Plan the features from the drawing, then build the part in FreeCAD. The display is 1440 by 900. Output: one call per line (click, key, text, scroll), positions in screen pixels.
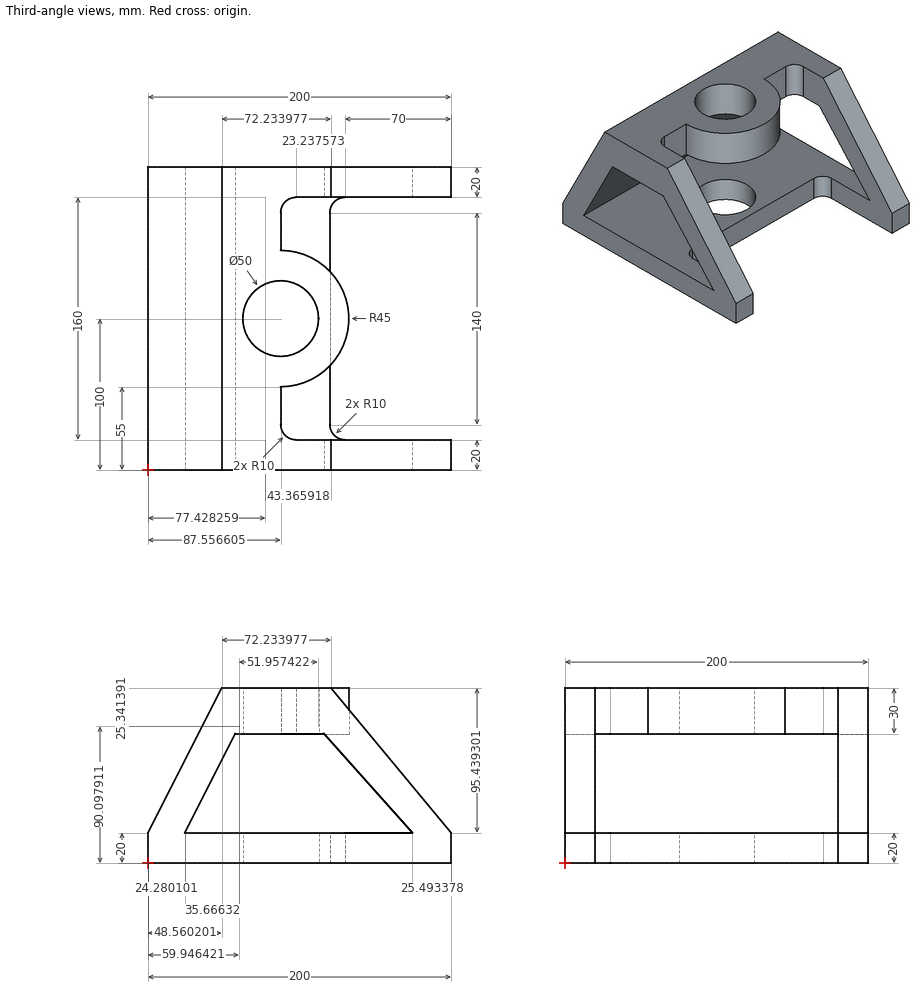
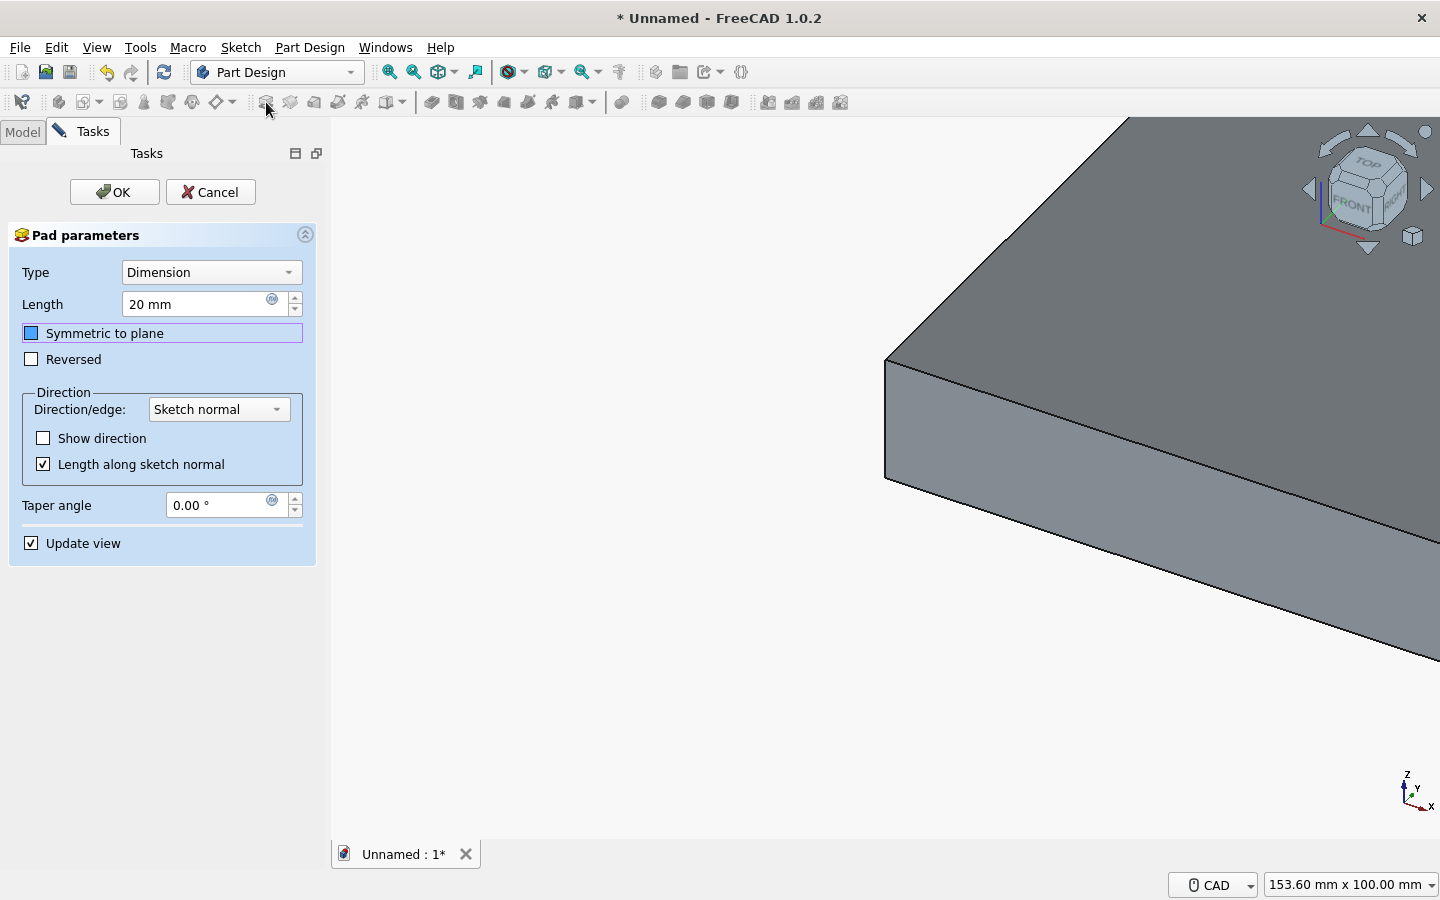
click(115, 192)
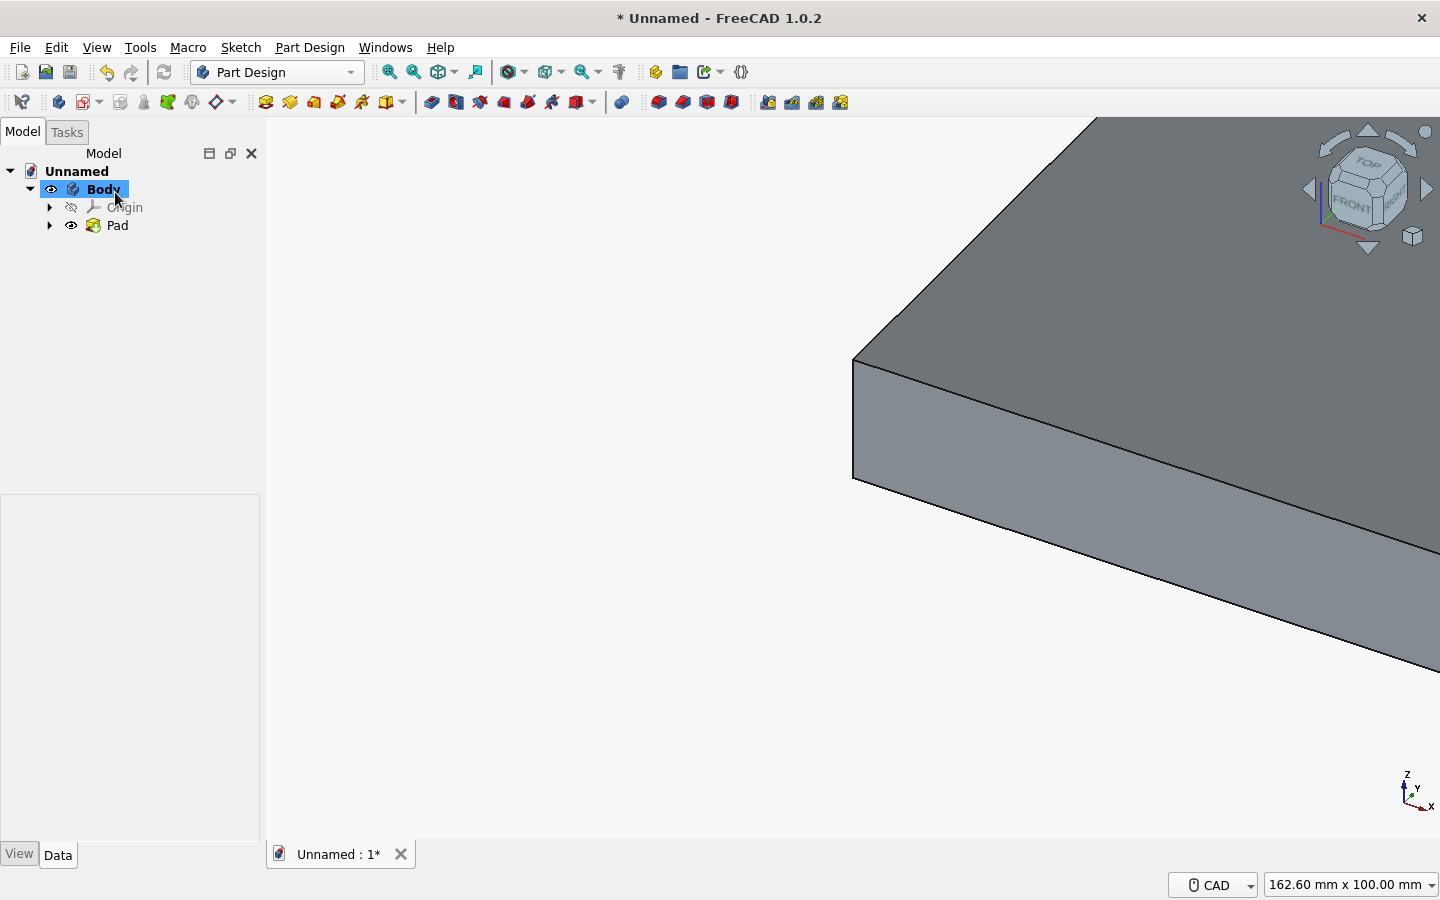
key(v)
key(f)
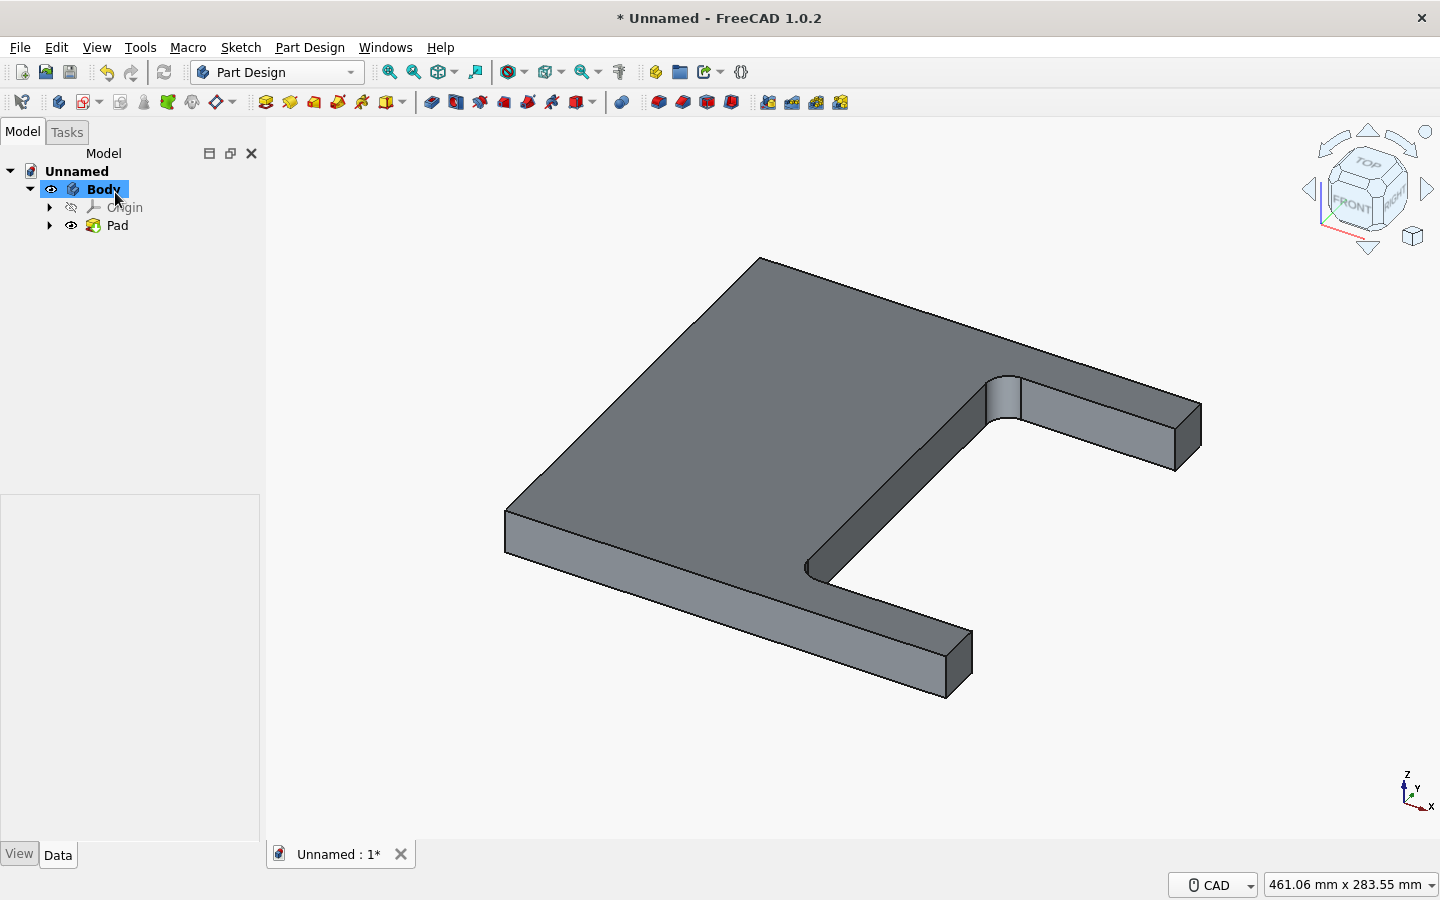
click(915, 666)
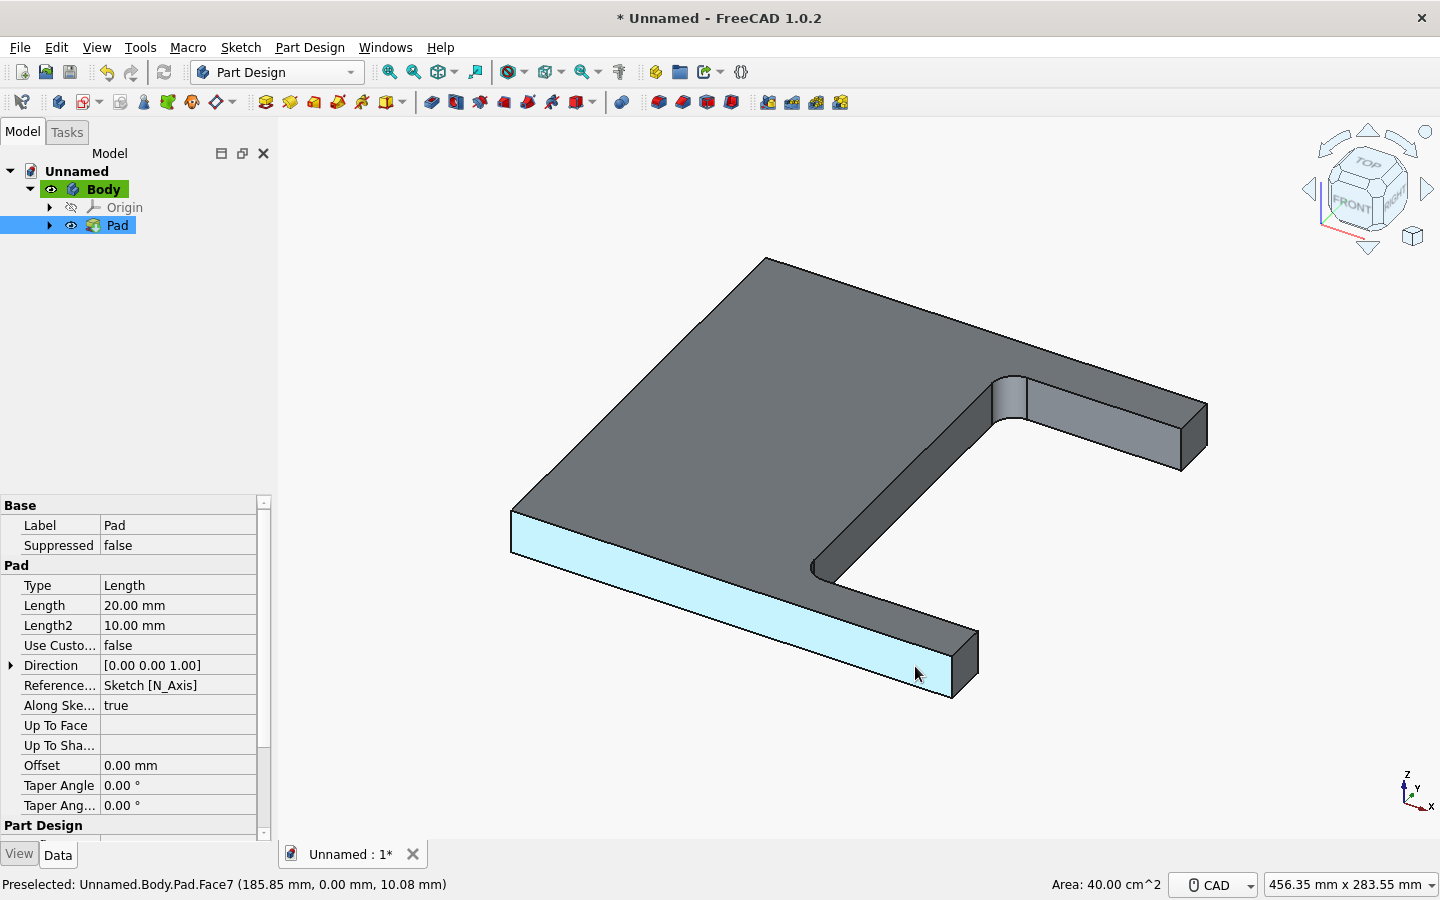
click(84, 102)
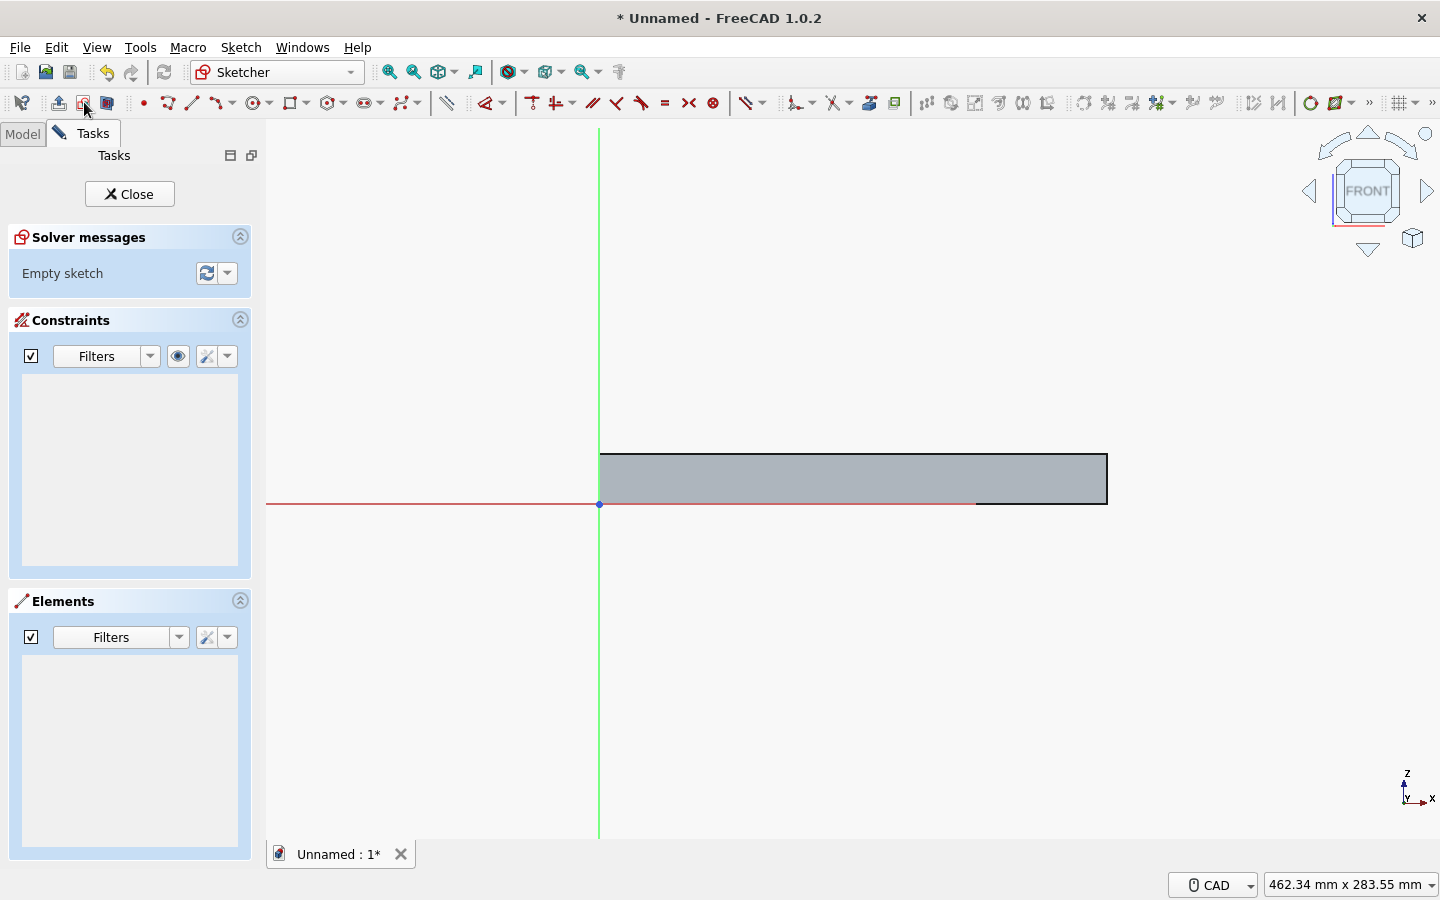
scroll(992, 147, up, 2)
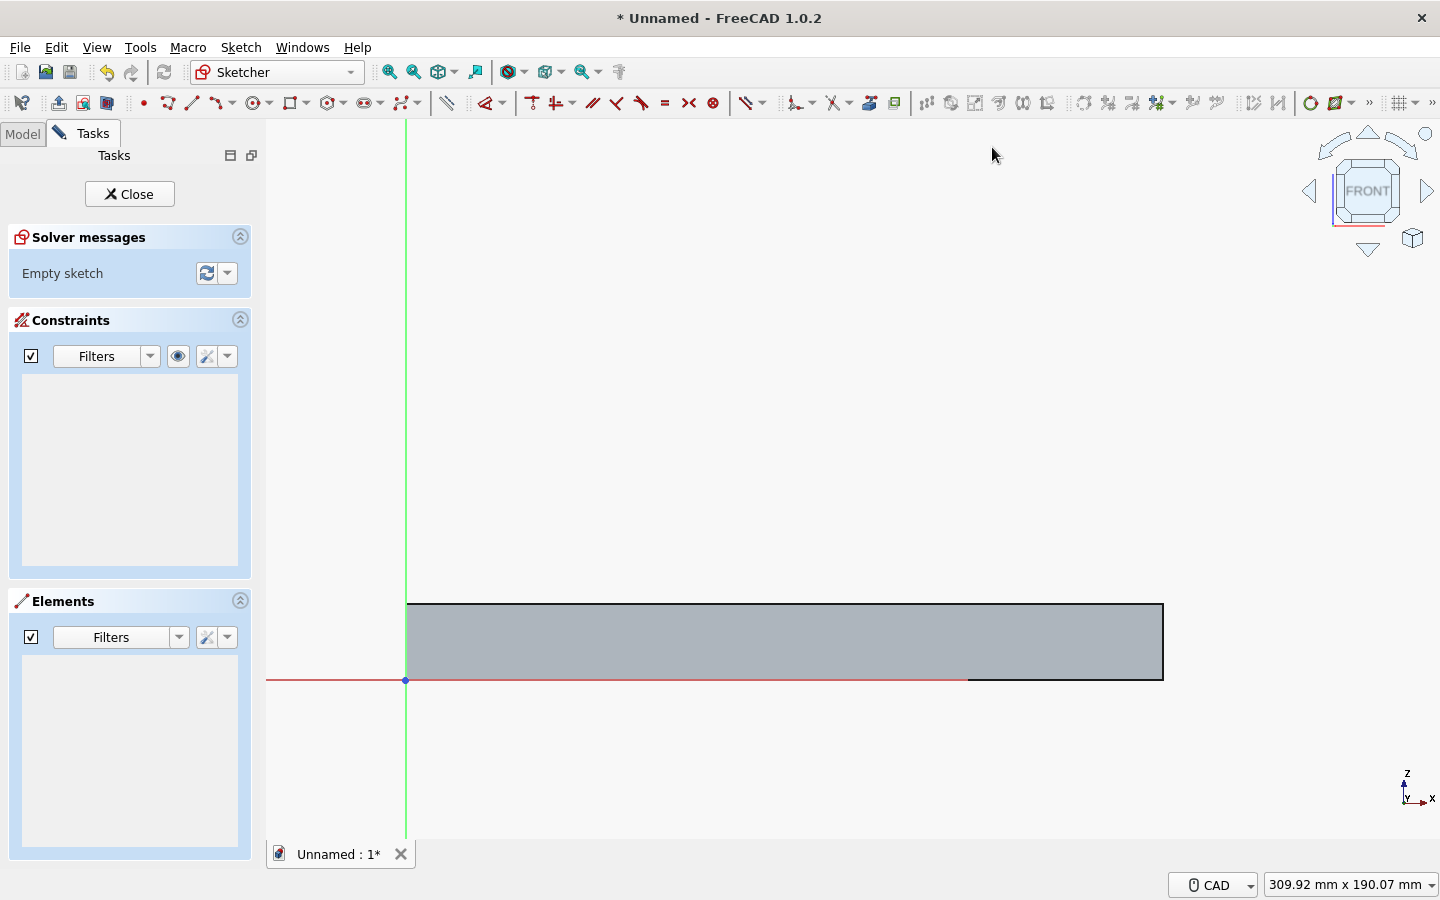
click(168, 104)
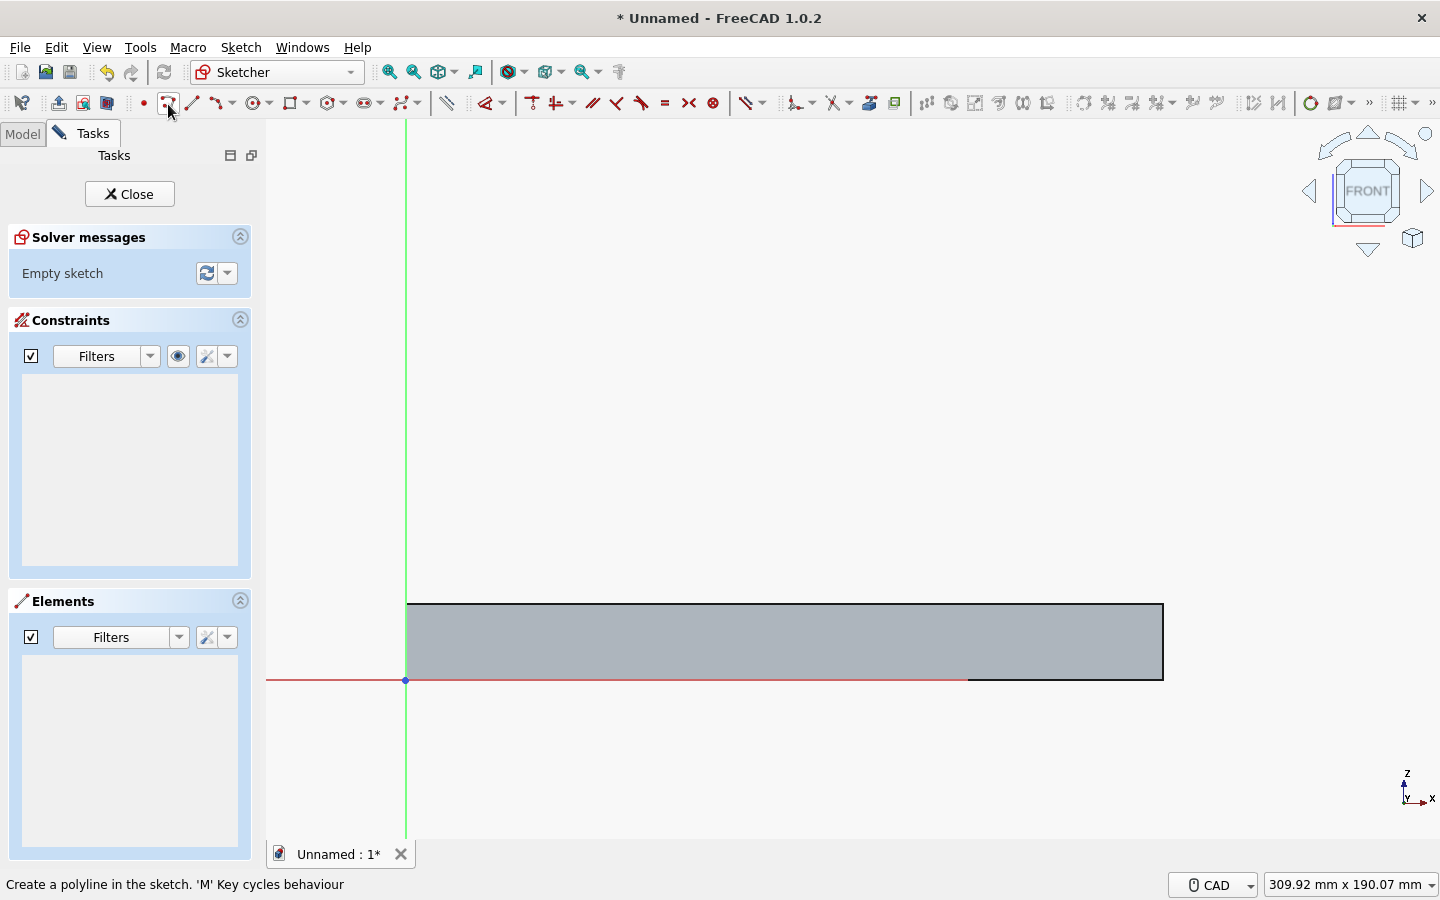
click(406, 604)
click(497, 604)
click(633, 339)
click(829, 339)
click(1067, 604)
click(1163, 604)
click(863, 243)
click(589, 243)
click(406, 605)
key(Escape)
key(Escape)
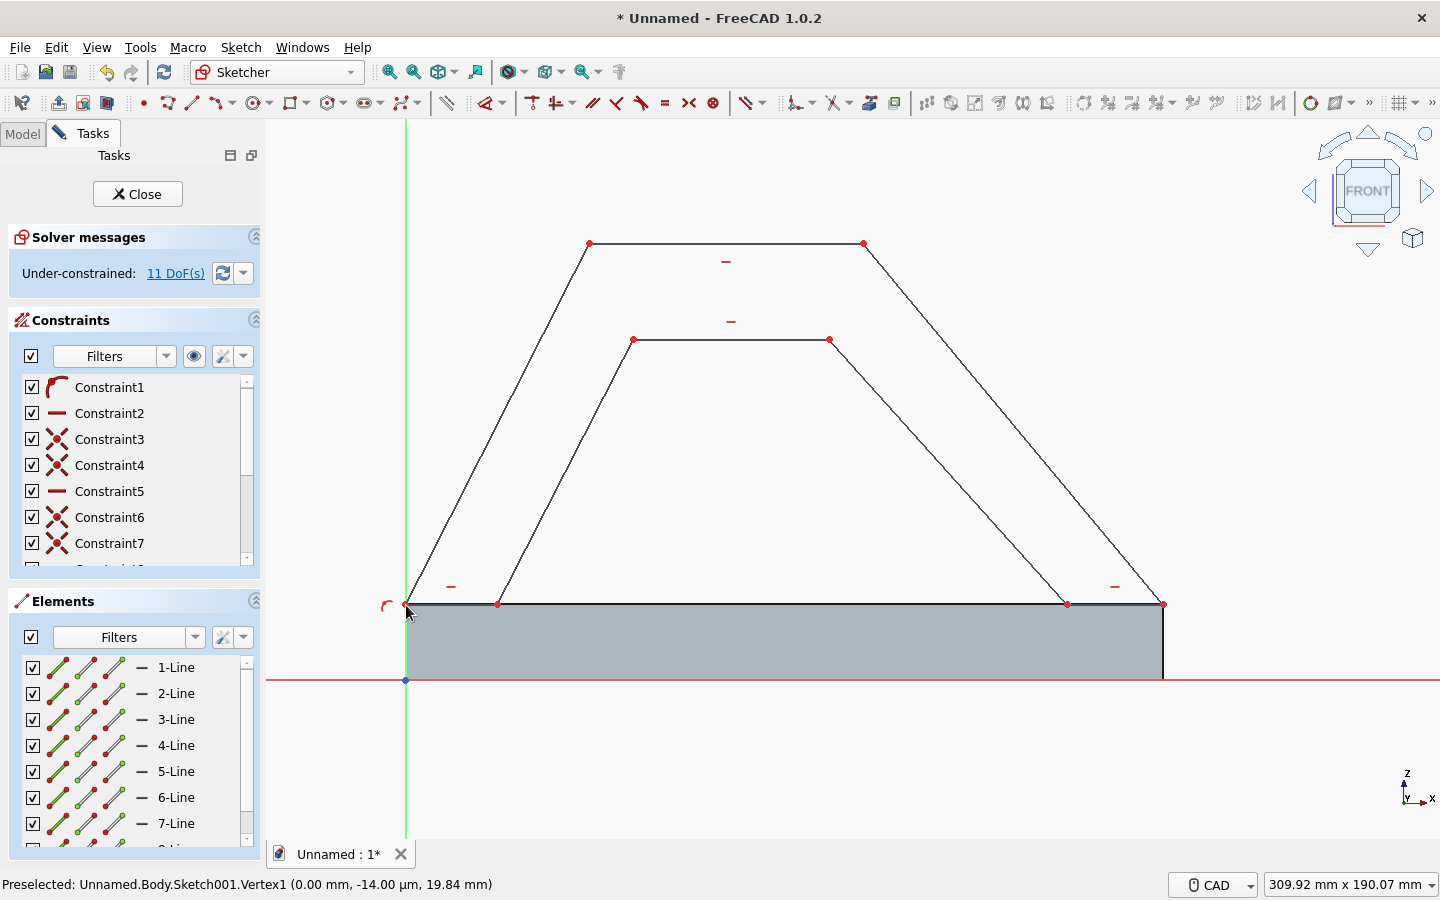
key(d)